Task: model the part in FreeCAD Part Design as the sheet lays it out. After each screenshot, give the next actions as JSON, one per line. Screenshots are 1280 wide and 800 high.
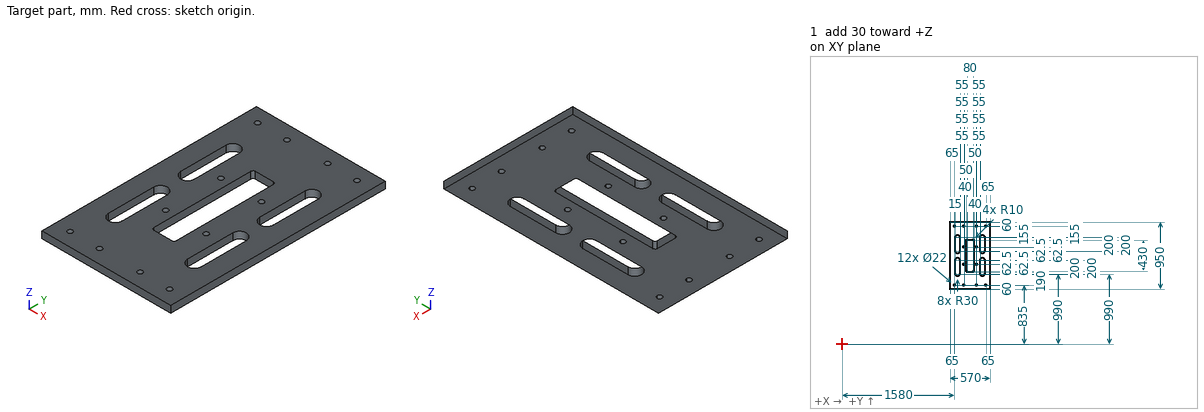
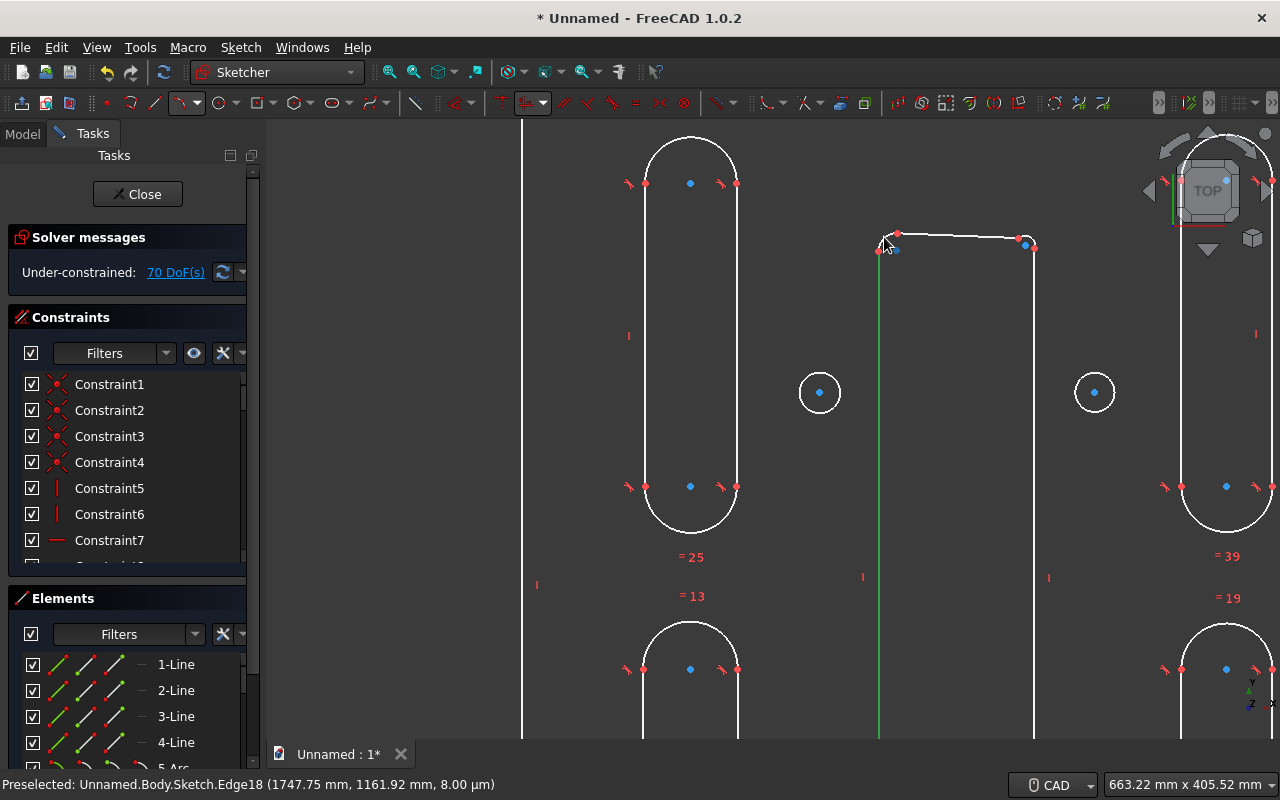
{"action": "left_click", "coordinate": [884, 238]}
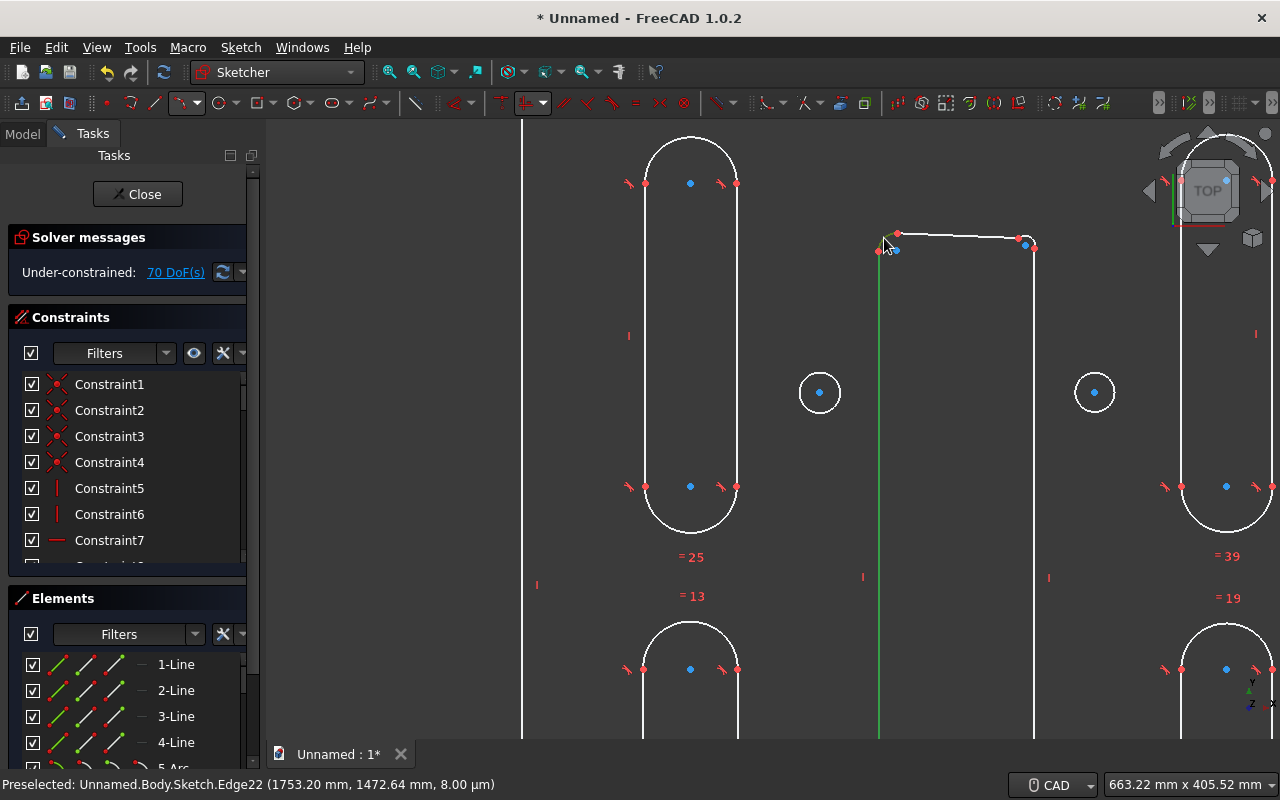
{"action": "left_click", "coordinate": [612, 104]}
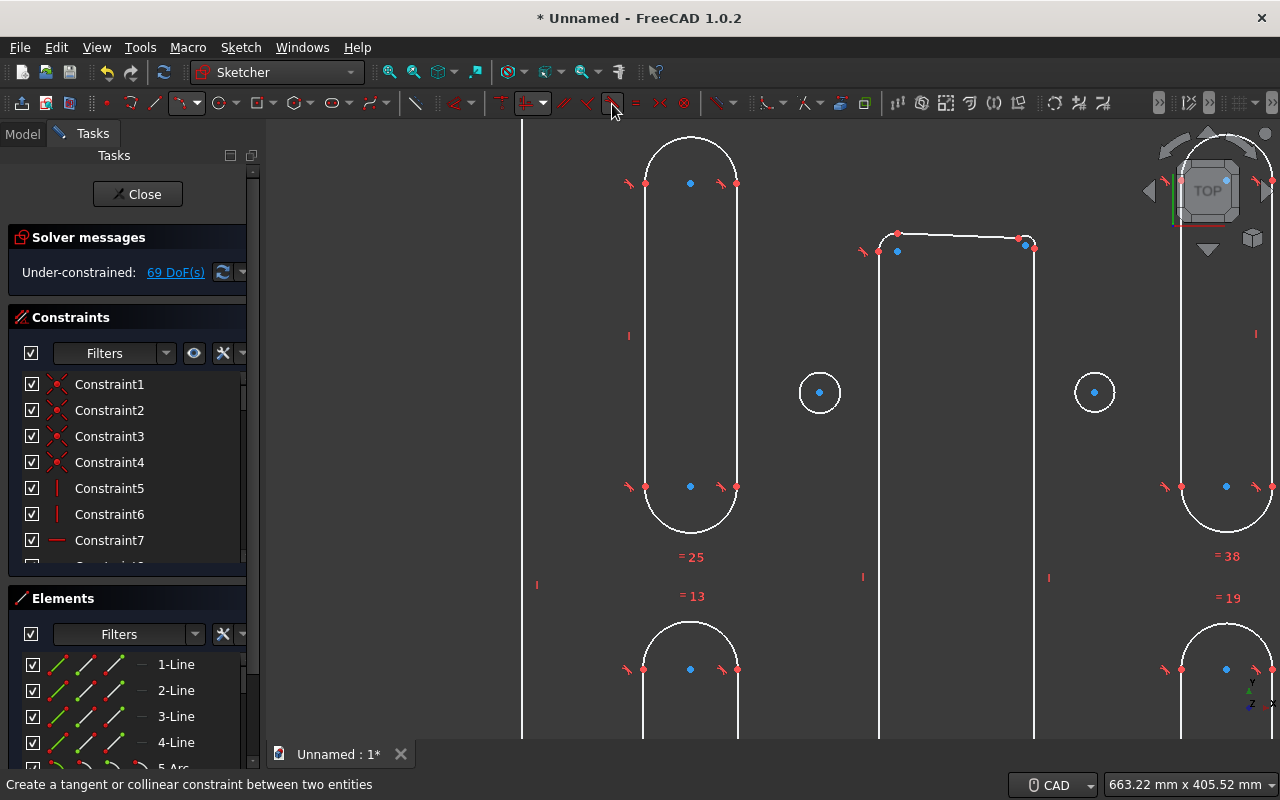
{"action": "left_click", "coordinate": [934, 235]}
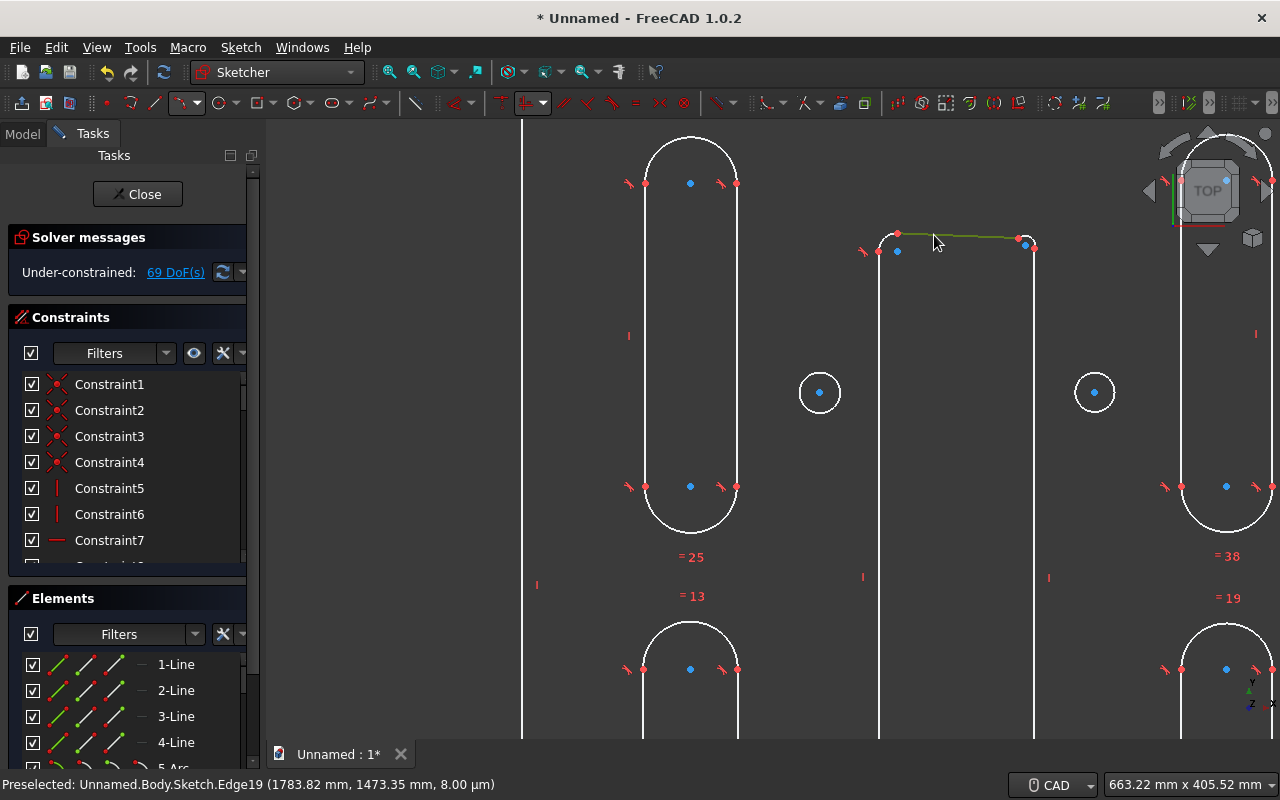
{"action": "left_click", "coordinate": [884, 239]}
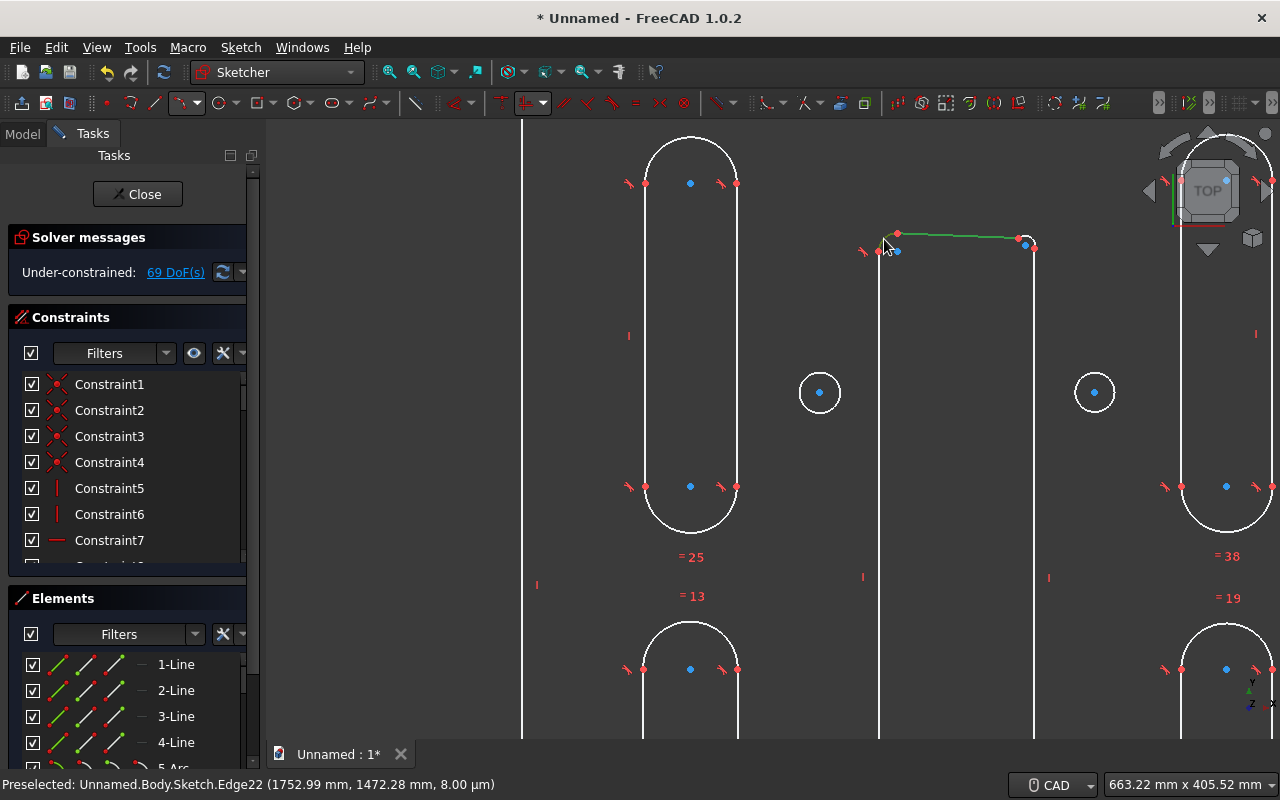
{"action": "left_click", "coordinate": [612, 104]}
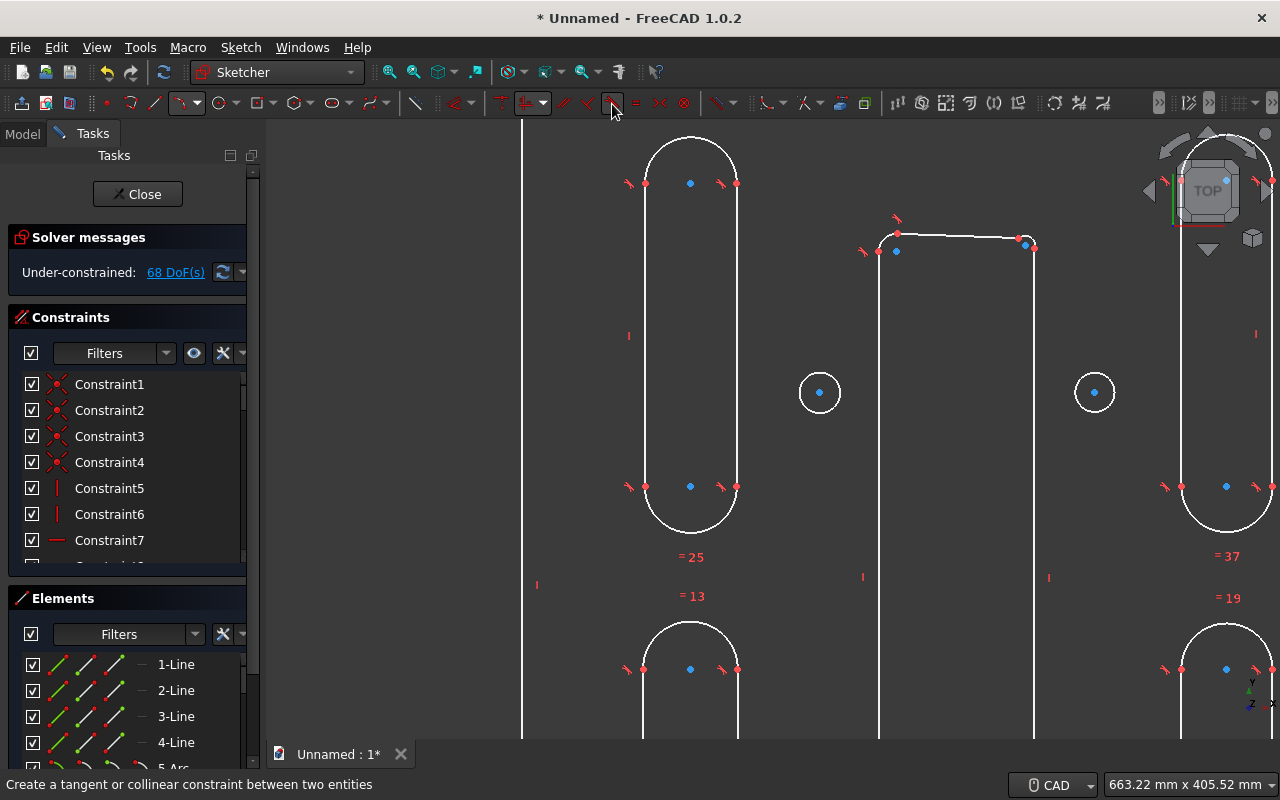
{"action": "left_click", "coordinate": [934, 235]}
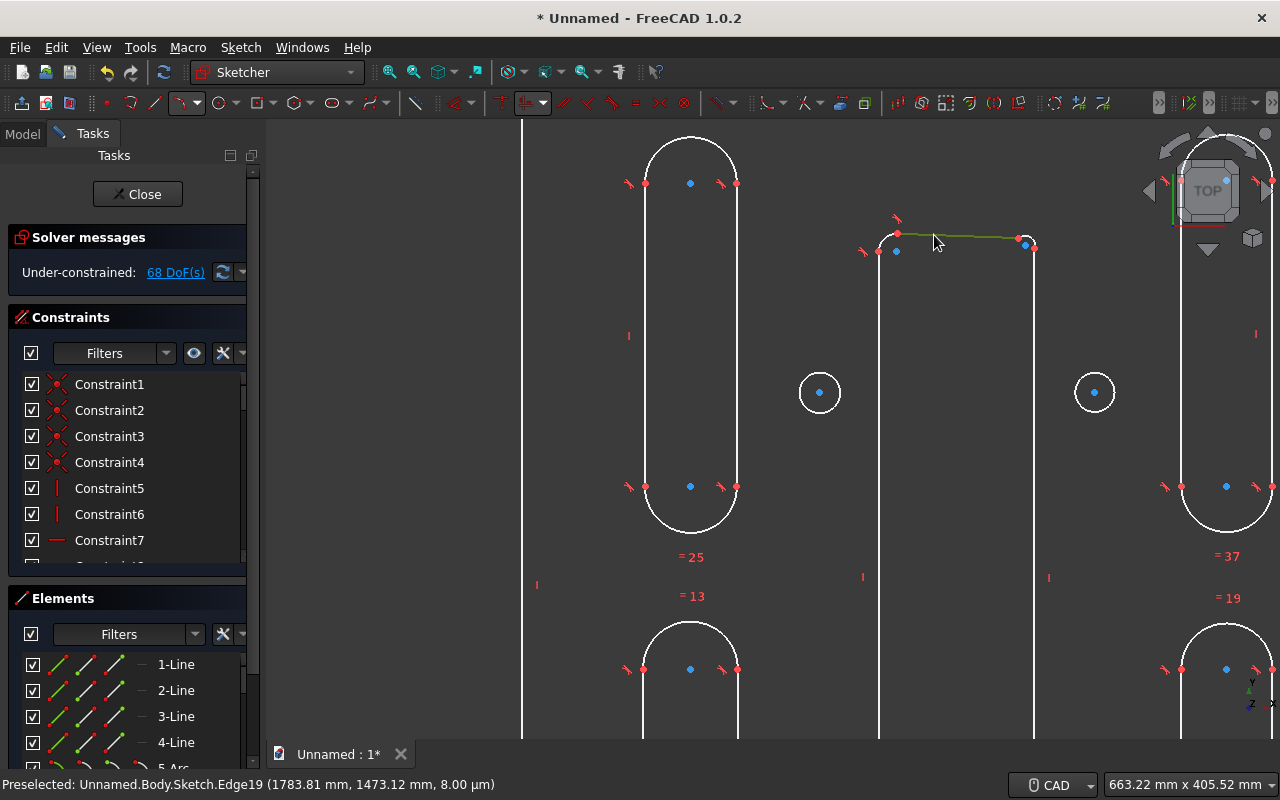
{"action": "scroll", "coordinate": [1031, 238], "scroll_direction": "up", "scroll_amount": 2}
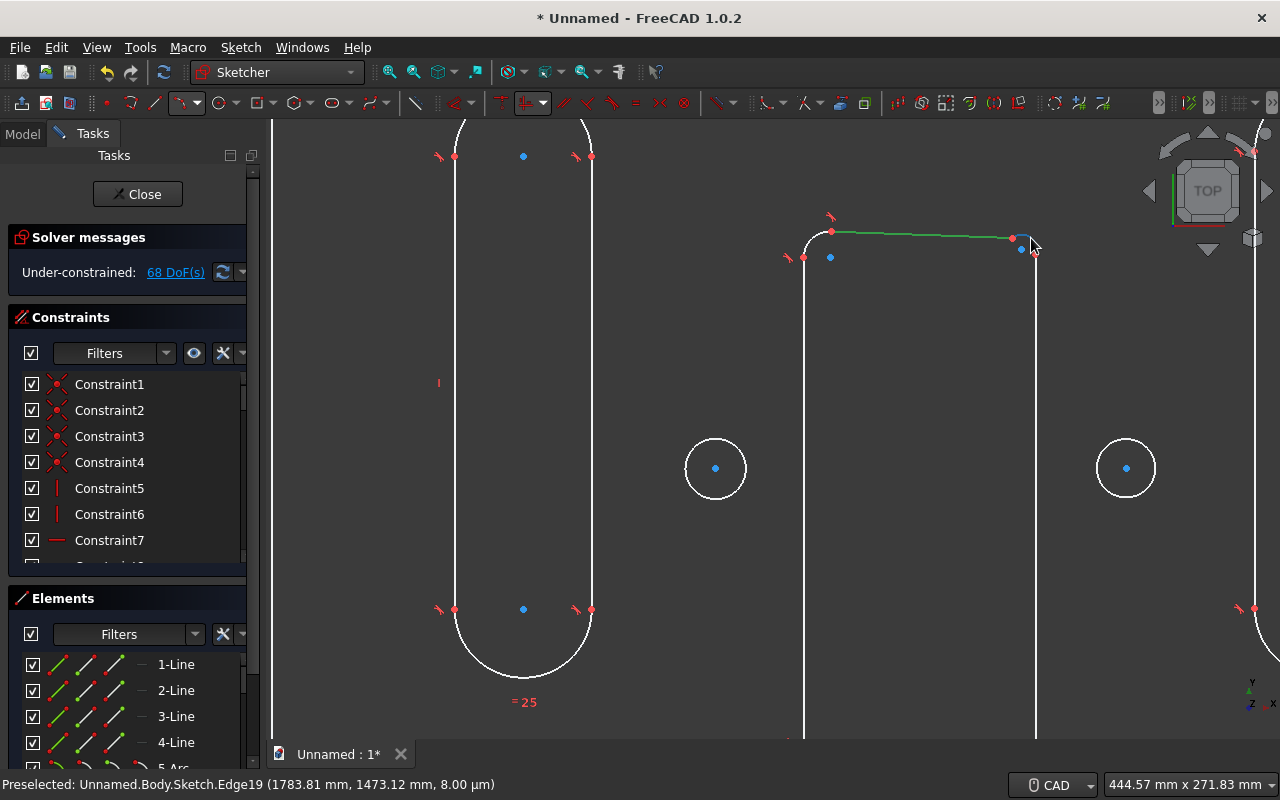
{"action": "left_click", "coordinate": [1030, 237]}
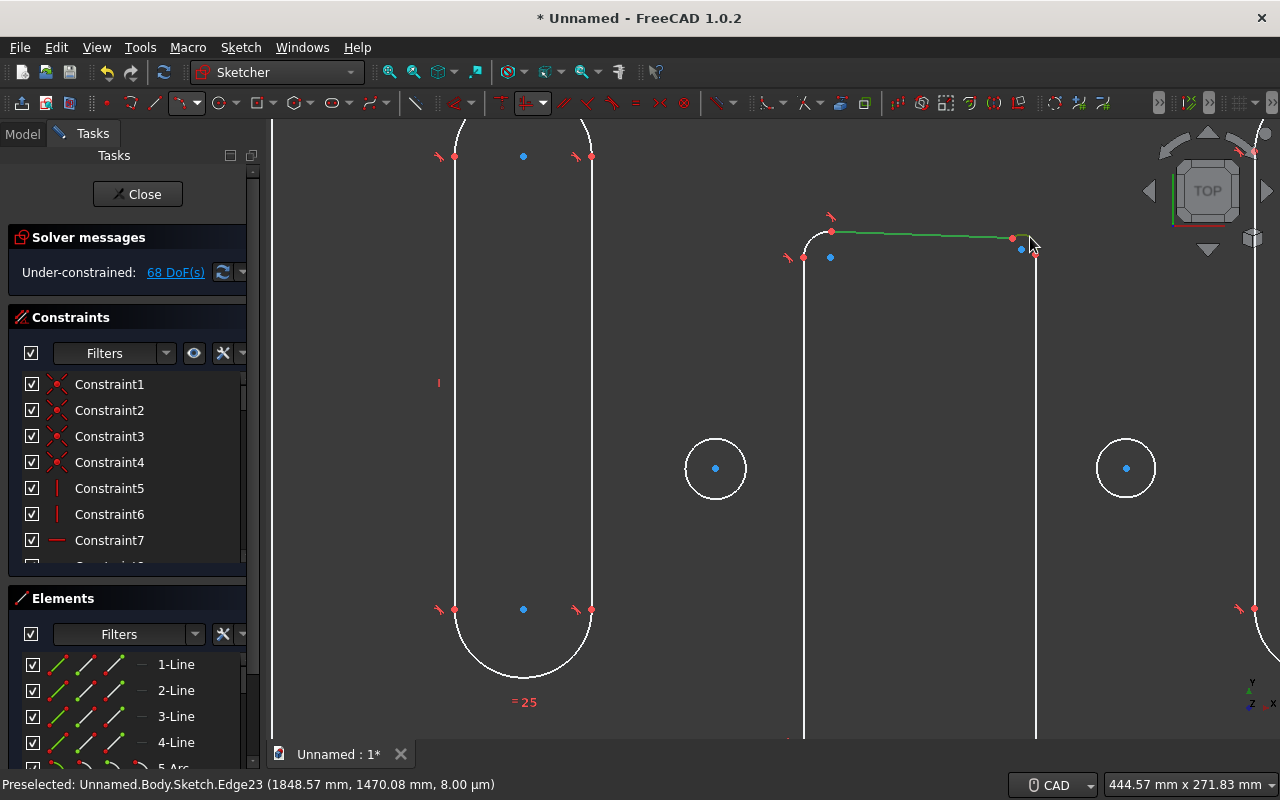
{"action": "left_click", "coordinate": [612, 104]}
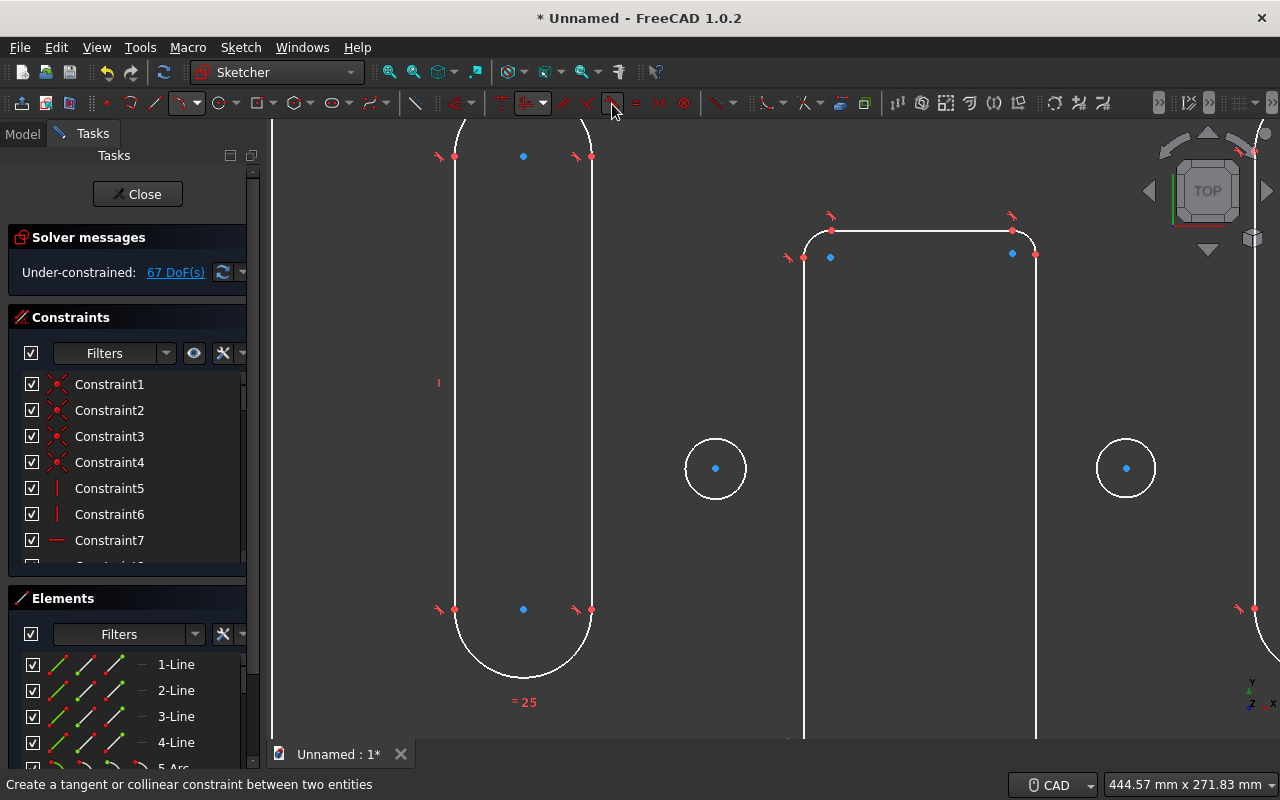
{"action": "scroll", "coordinate": [893, 280], "scroll_direction": "down", "scroll_amount": 11}